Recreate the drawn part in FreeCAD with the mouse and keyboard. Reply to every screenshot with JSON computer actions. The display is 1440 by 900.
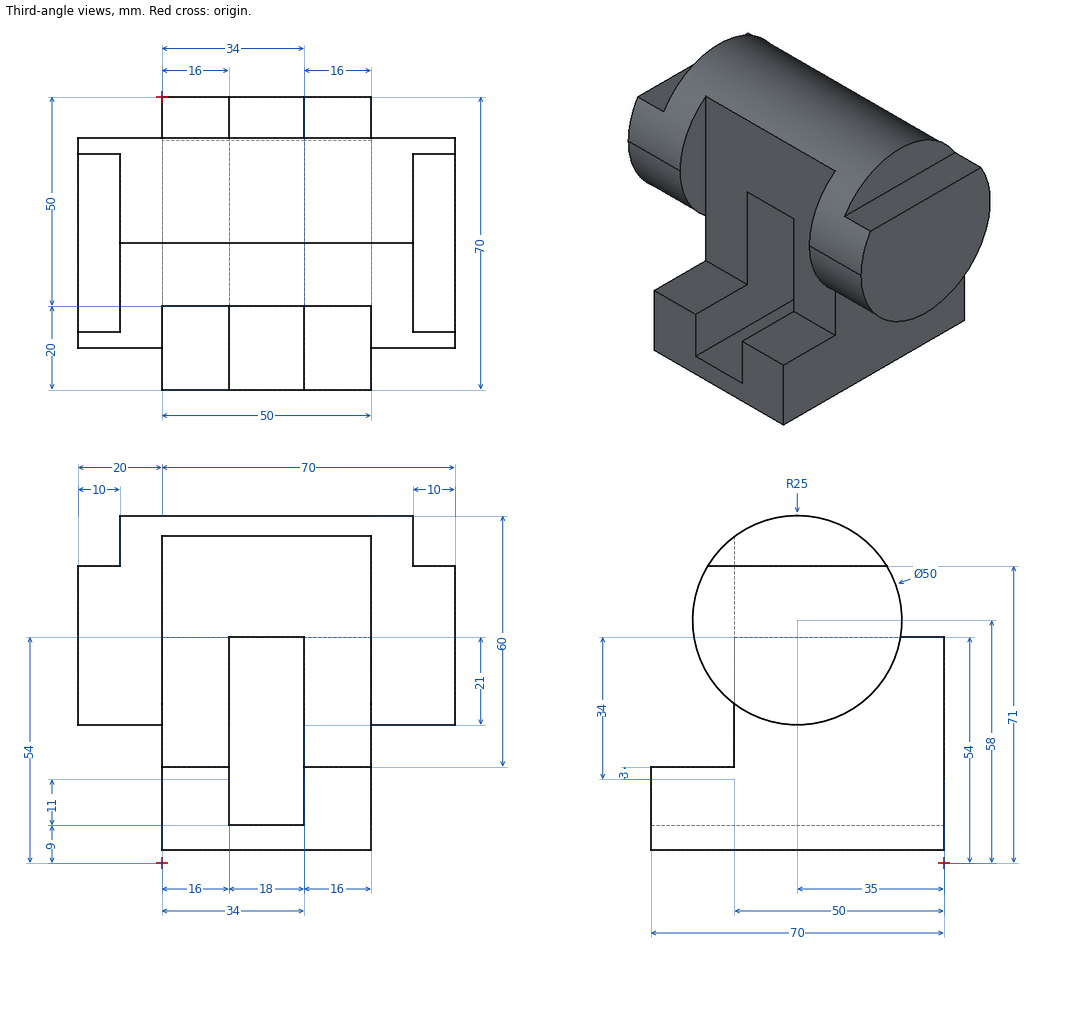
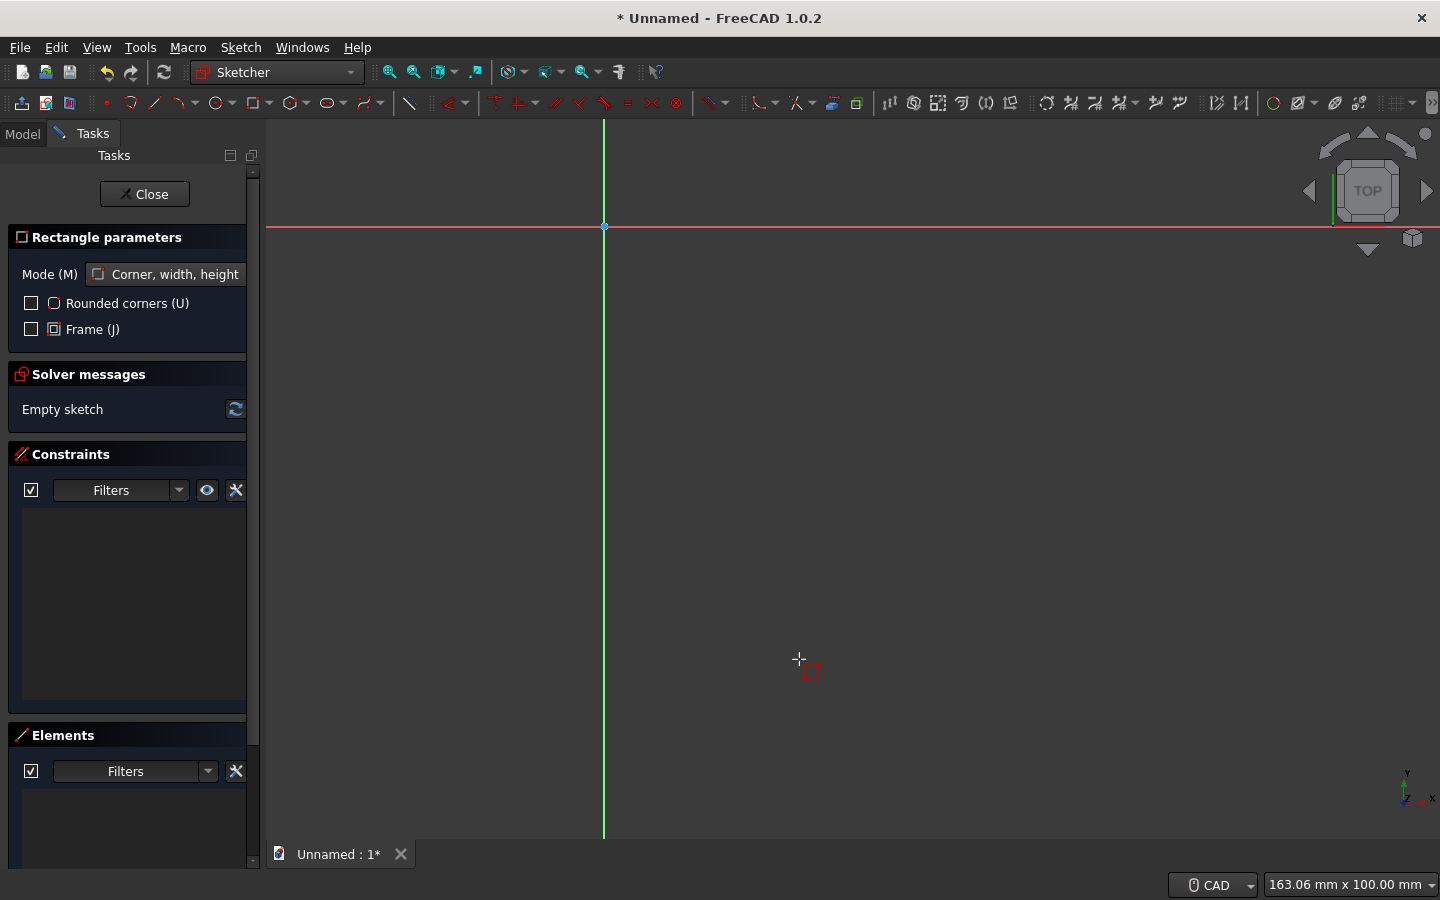
{"action": "left_click", "coordinate": [604, 227]}
{"action": "mouse_move", "coordinate": [964, 731]}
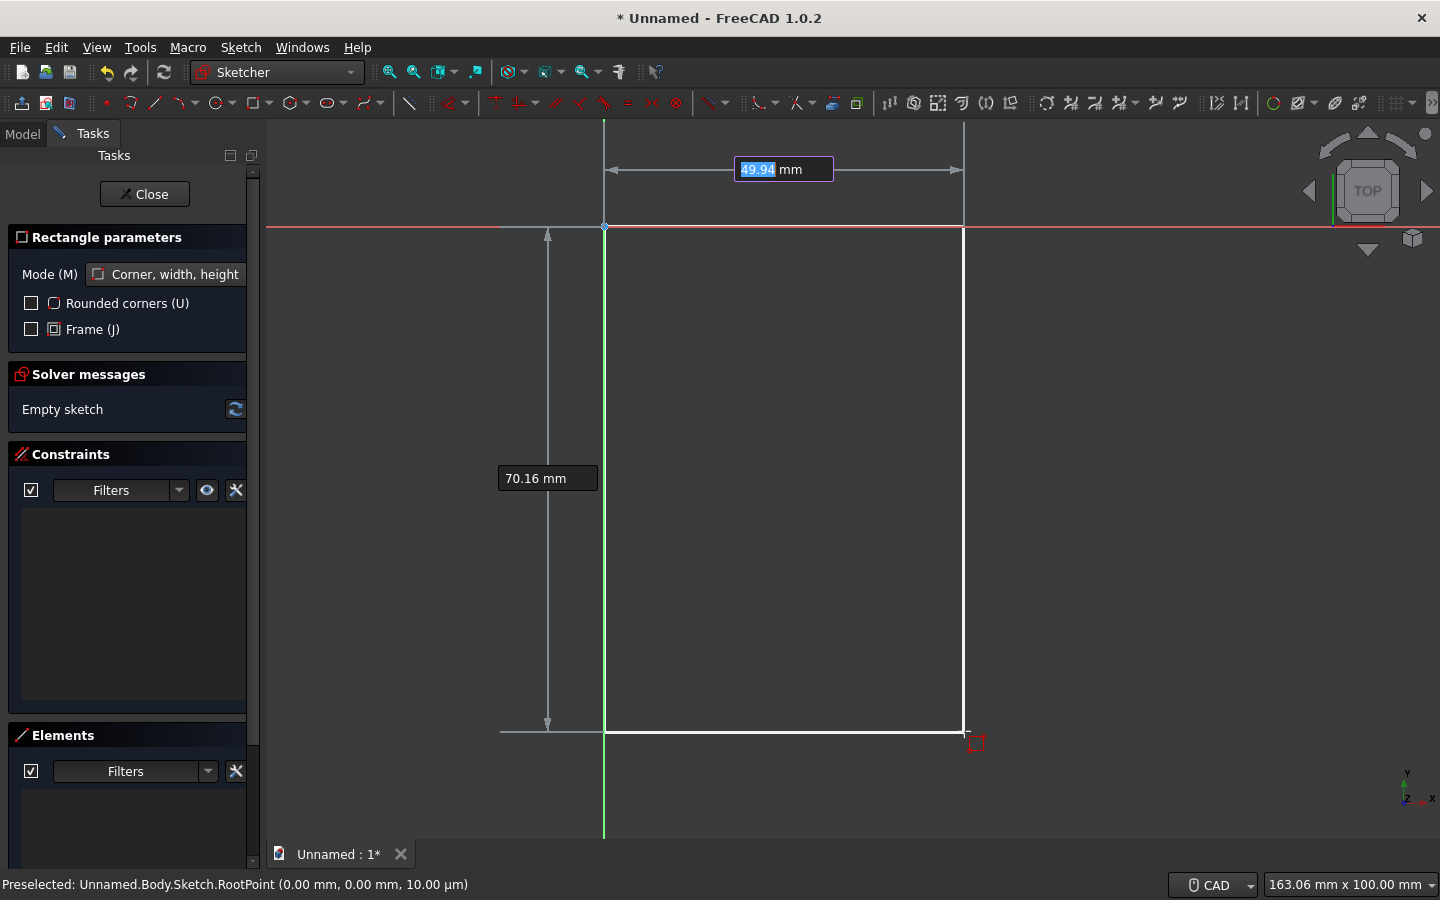
{"action": "type", "text": "50"}
{"action": "key", "text": "Tab"}
{"action": "type", "text": "70"}
{"action": "key", "text": "Return"}
{"action": "key", "text": "Escape"}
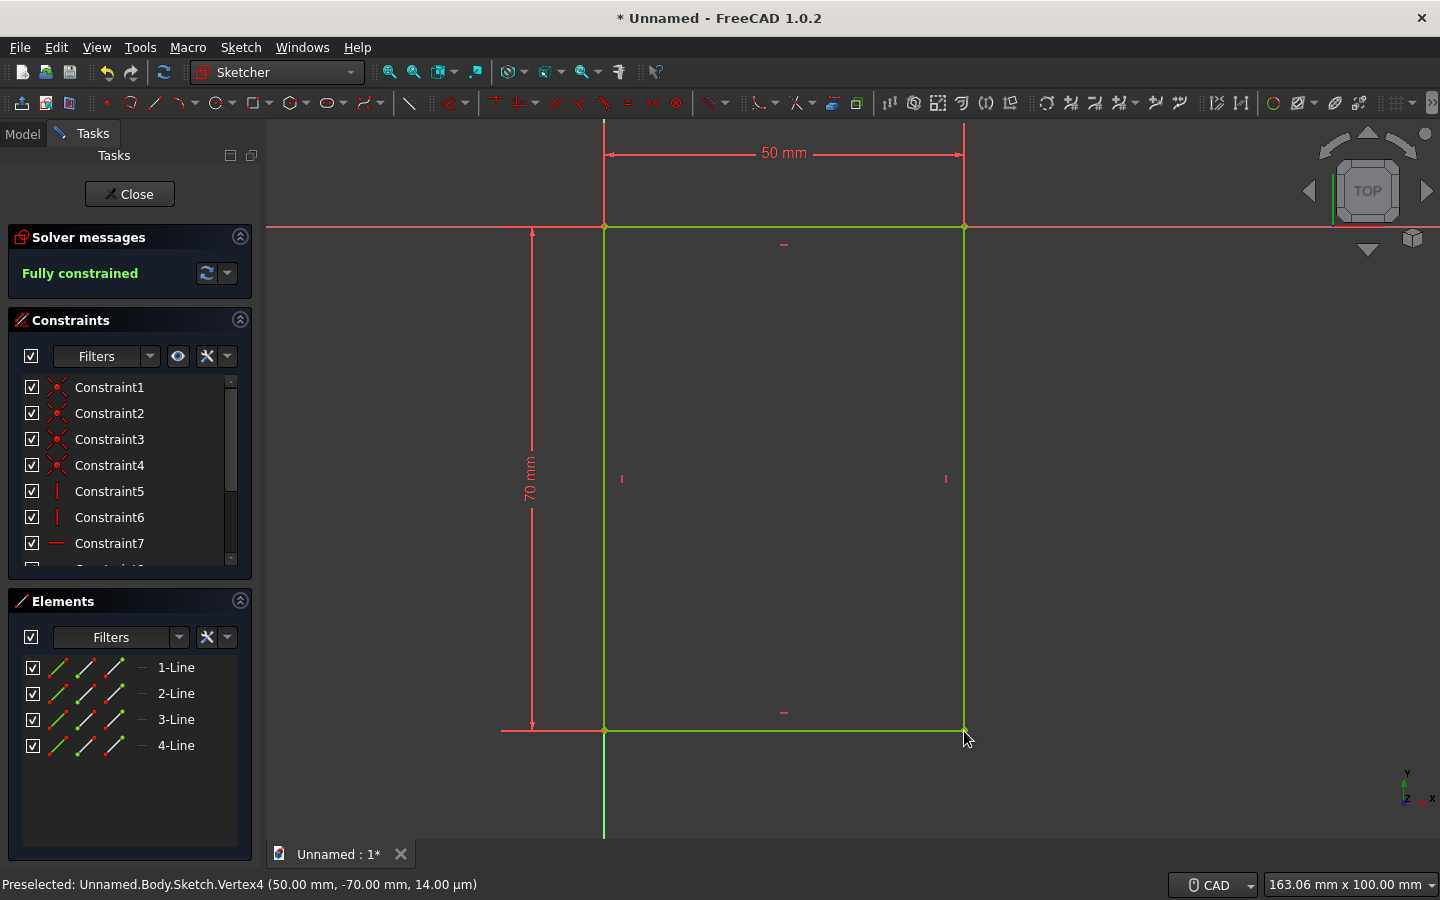
{"action": "left_click", "coordinate": [130, 194]}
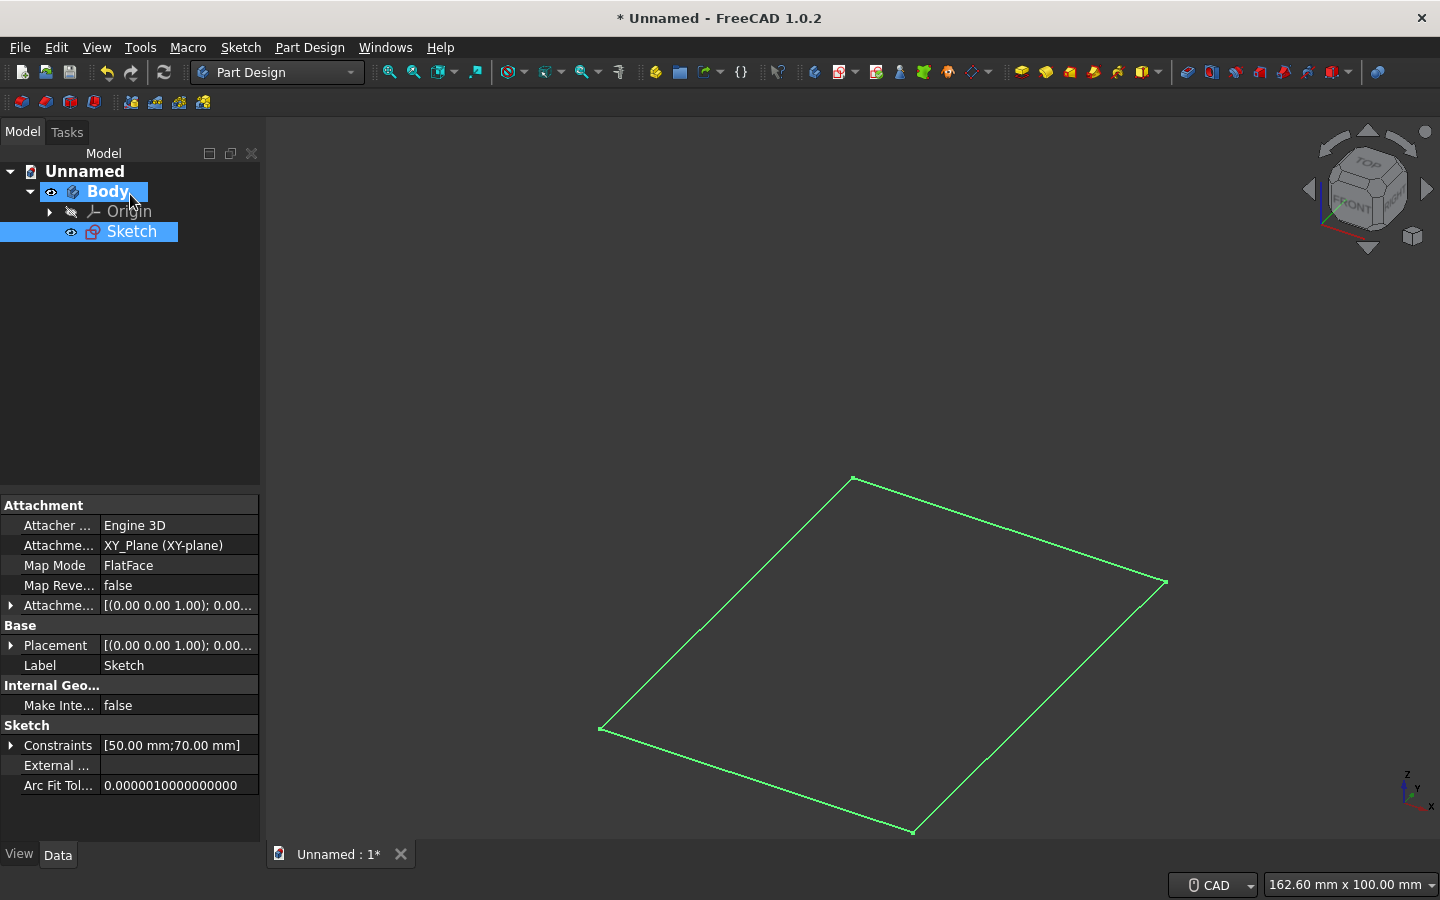
{"action": "left_click", "coordinate": [1022, 72]}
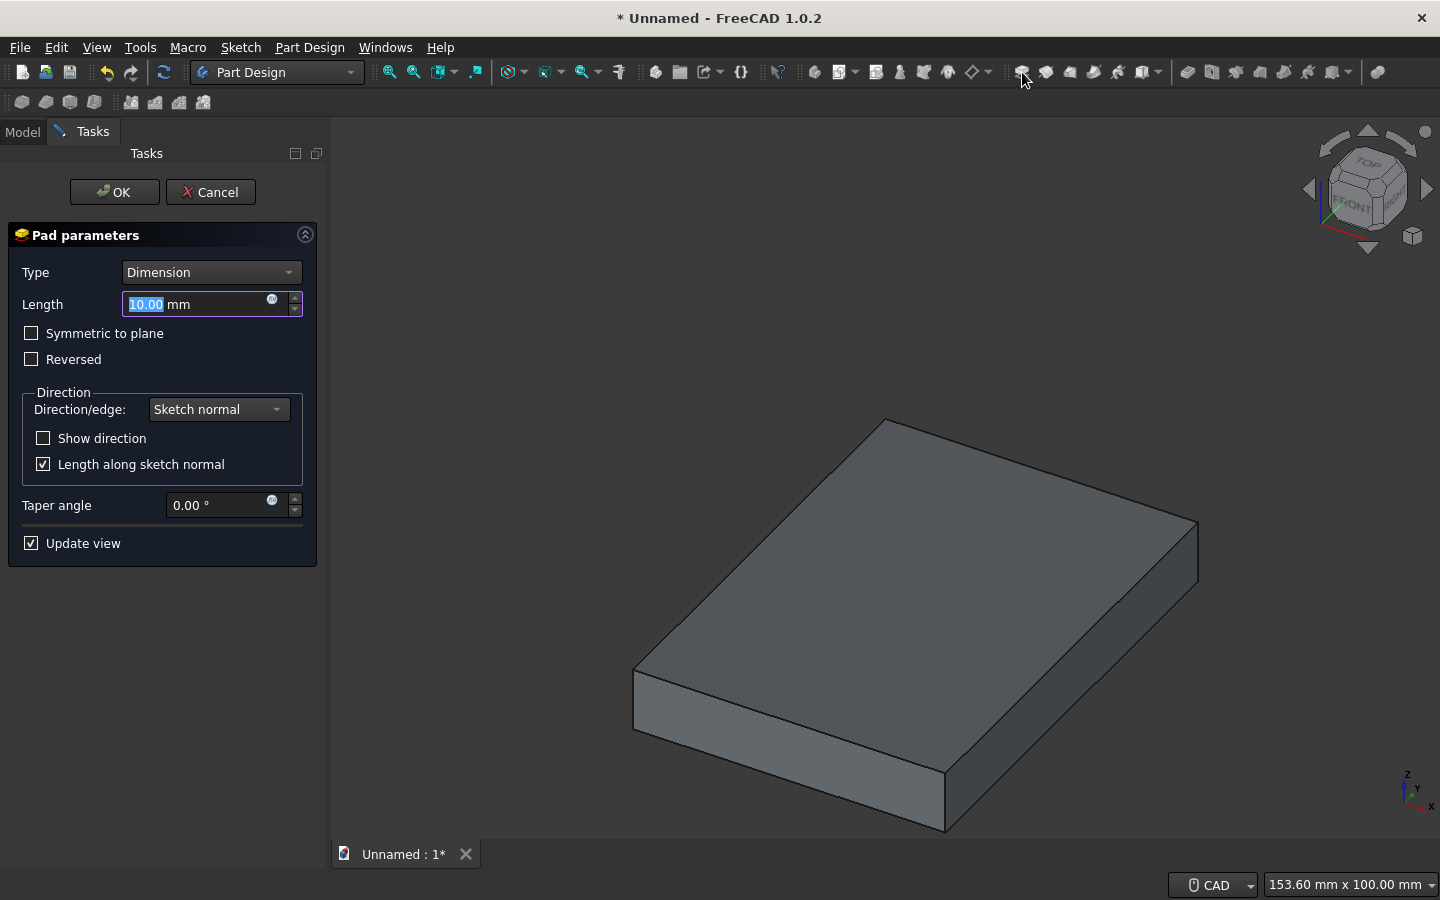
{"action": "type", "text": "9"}
{"action": "key", "text": "Tab"}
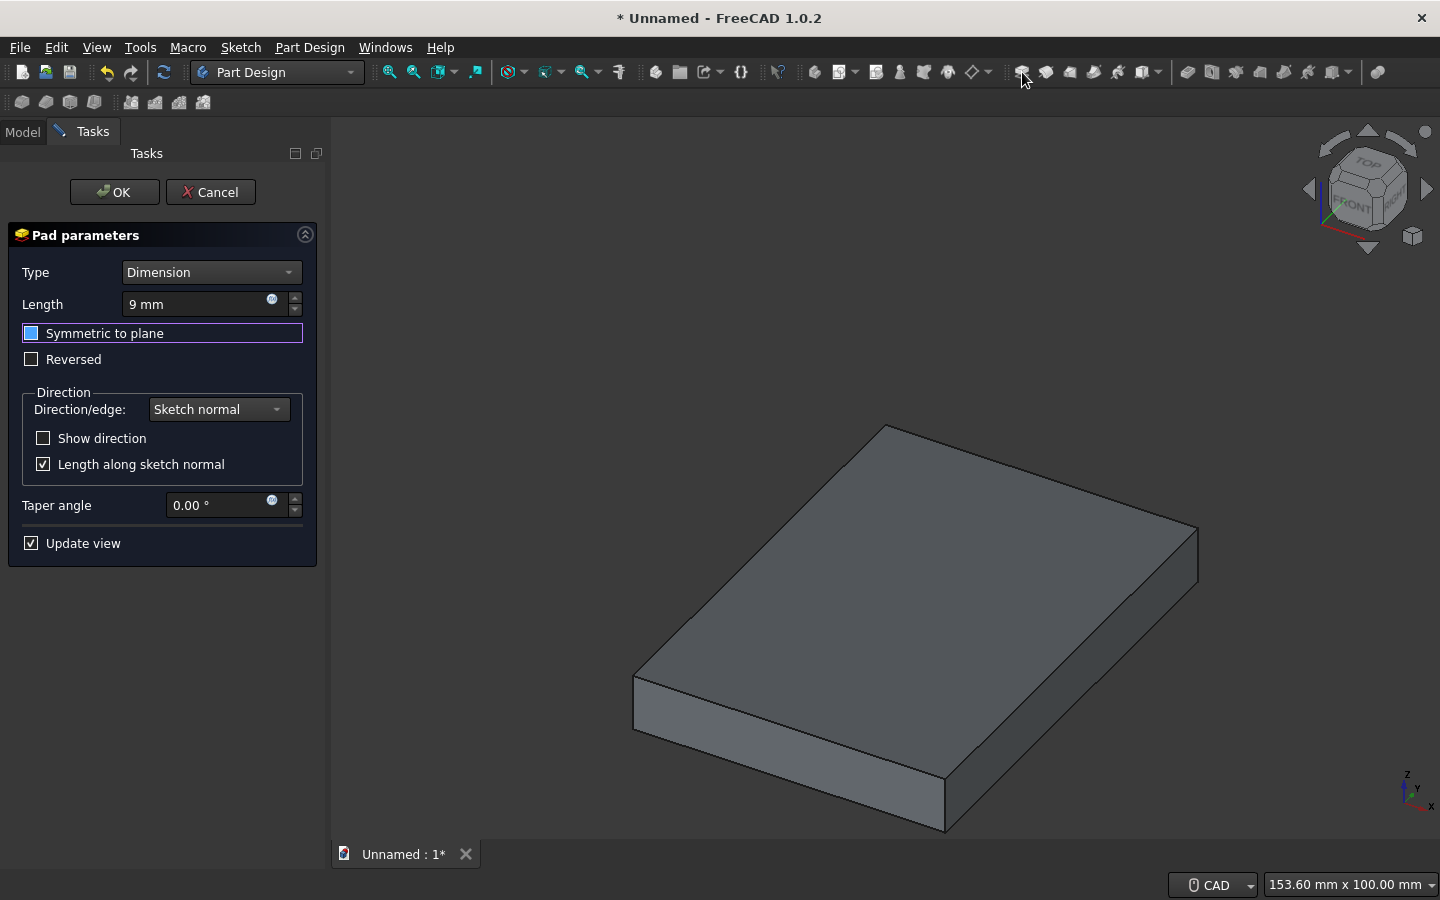
{"action": "left_click", "coordinate": [115, 192]}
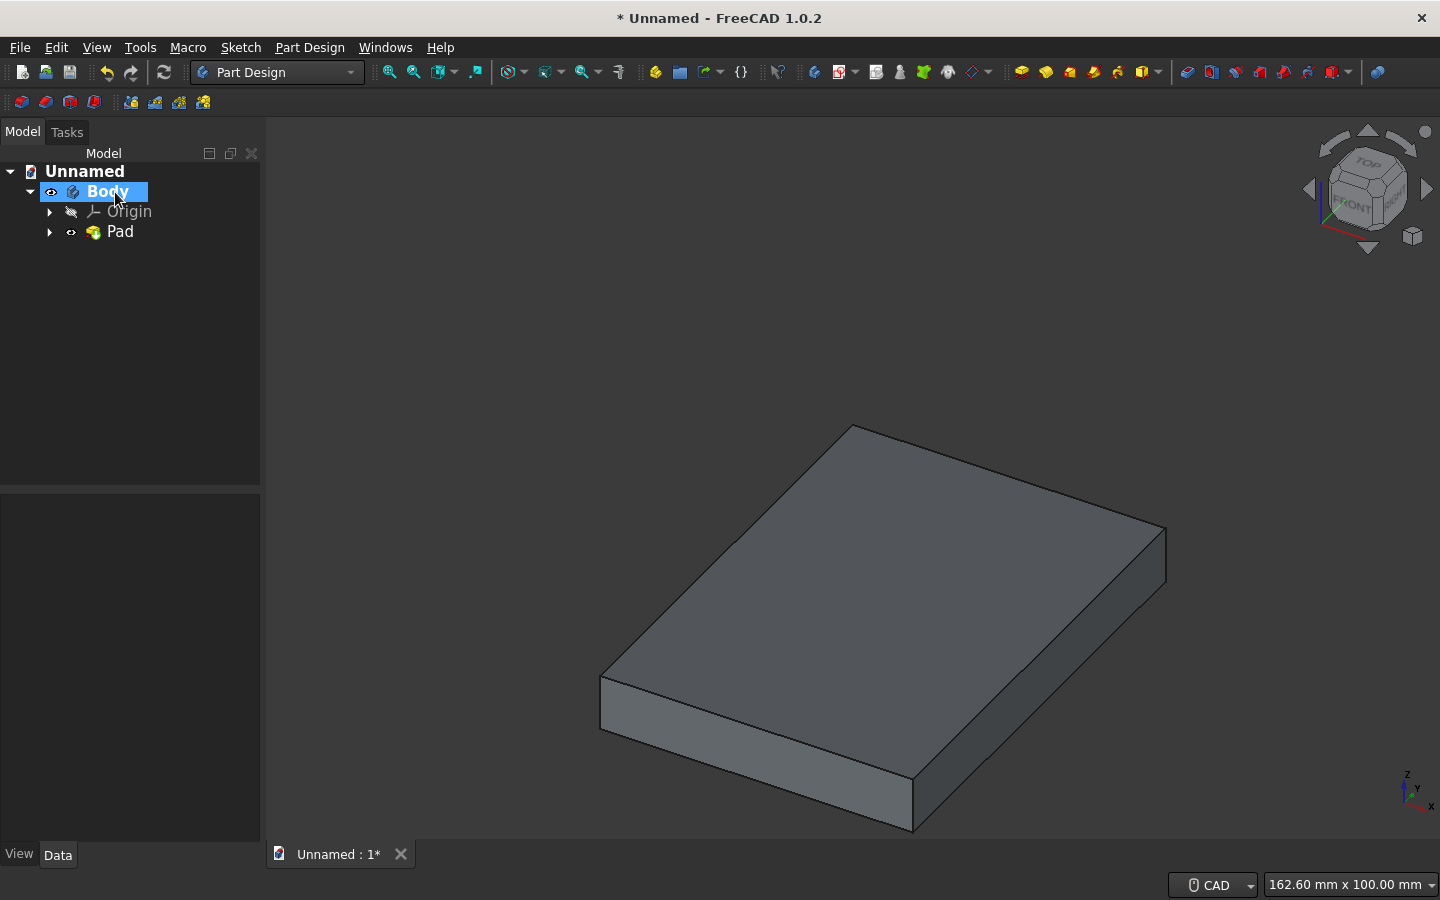
{"action": "left_click", "coordinate": [846, 783]}